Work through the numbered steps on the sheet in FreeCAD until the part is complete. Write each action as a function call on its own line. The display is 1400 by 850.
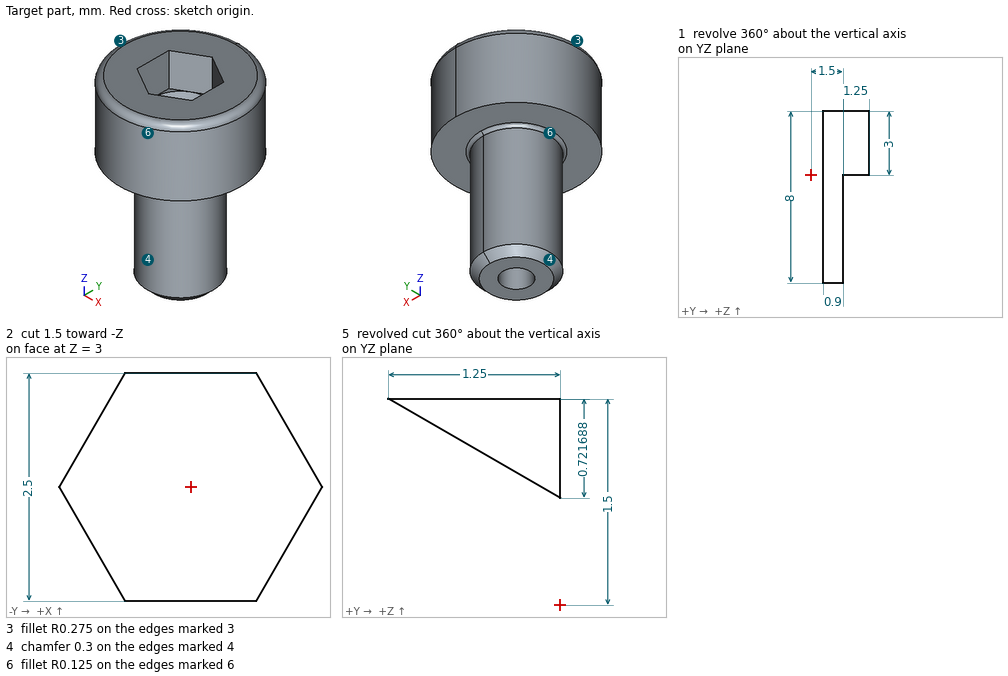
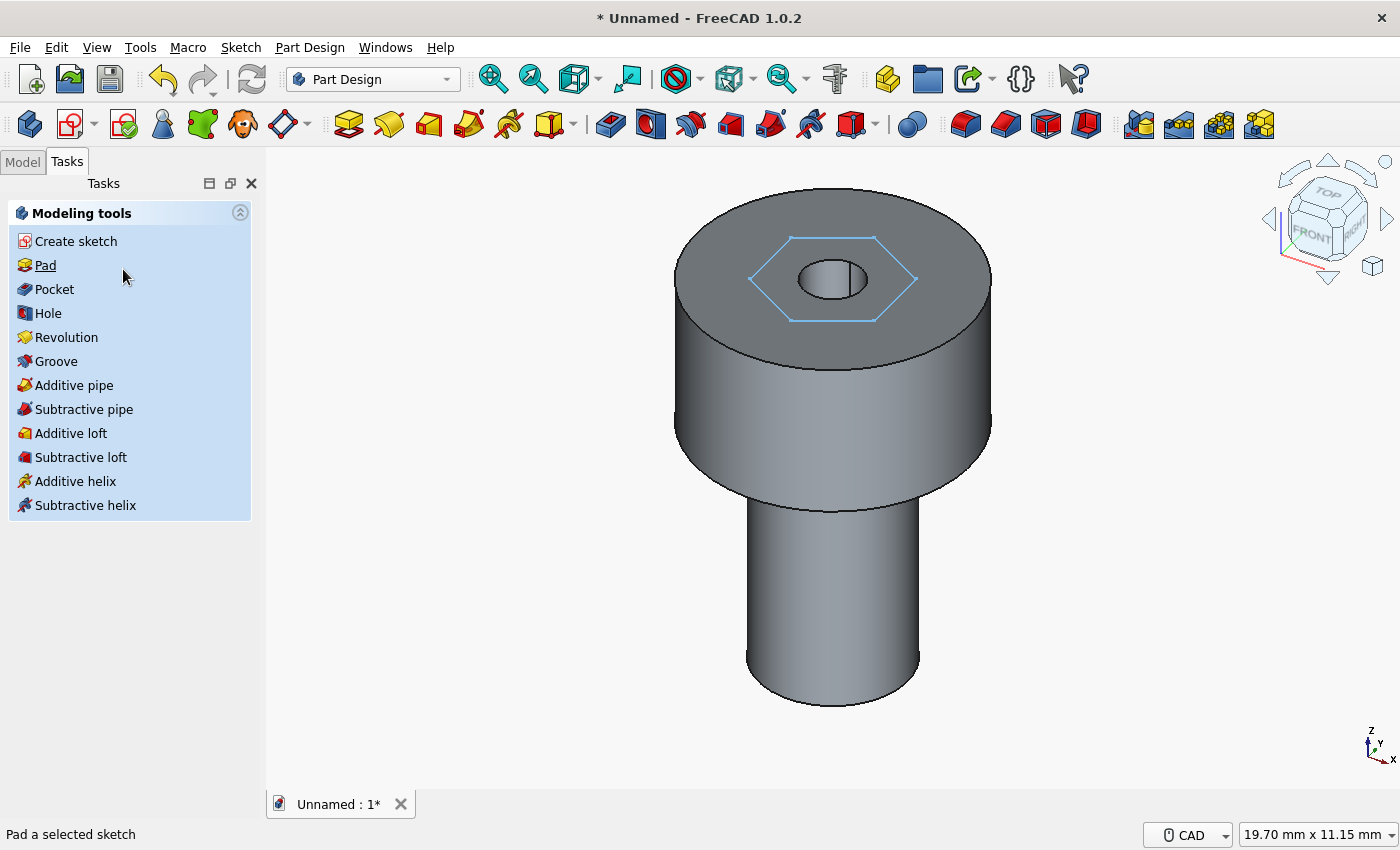
click(612, 124)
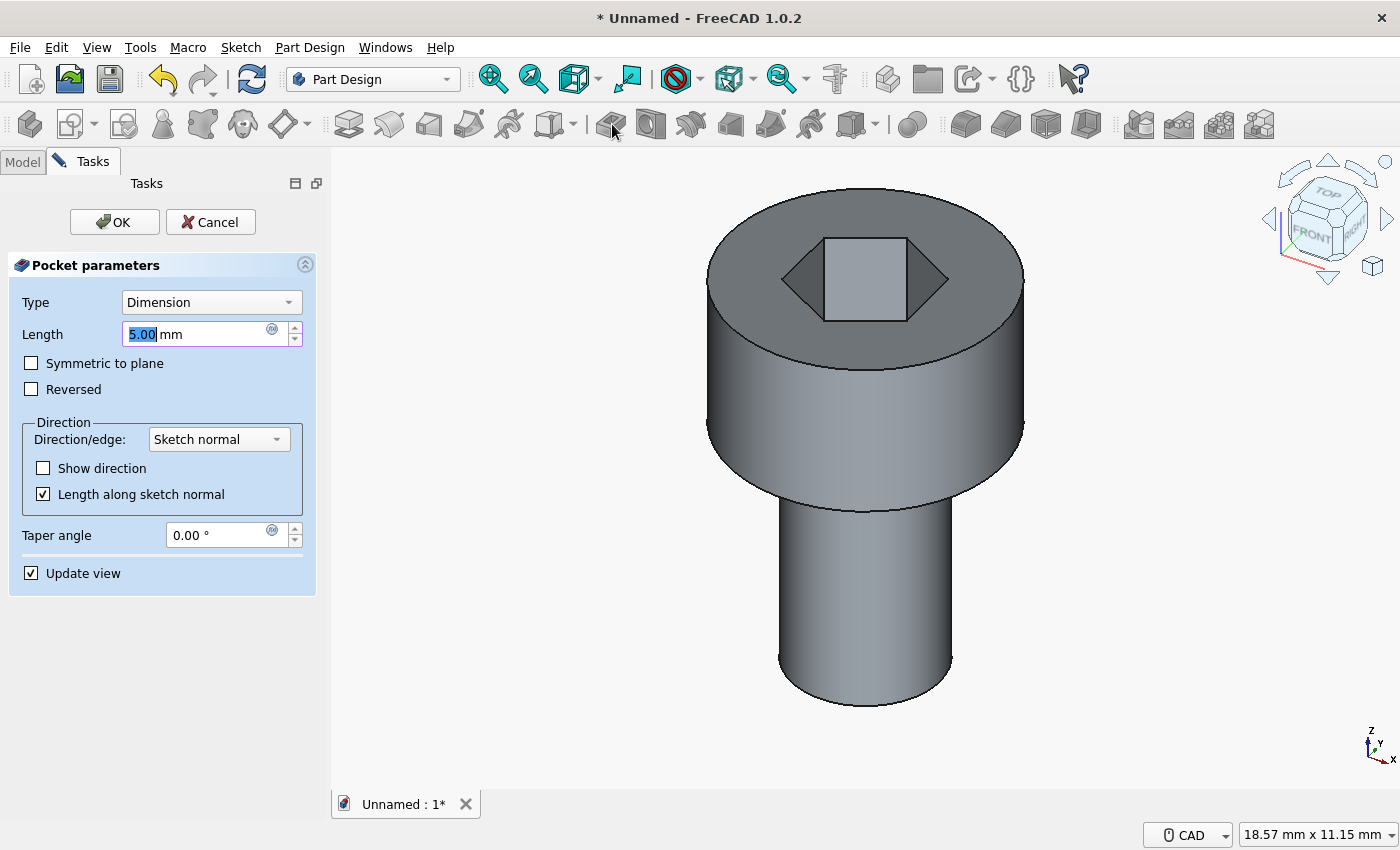
text(1.5)
key(Tab)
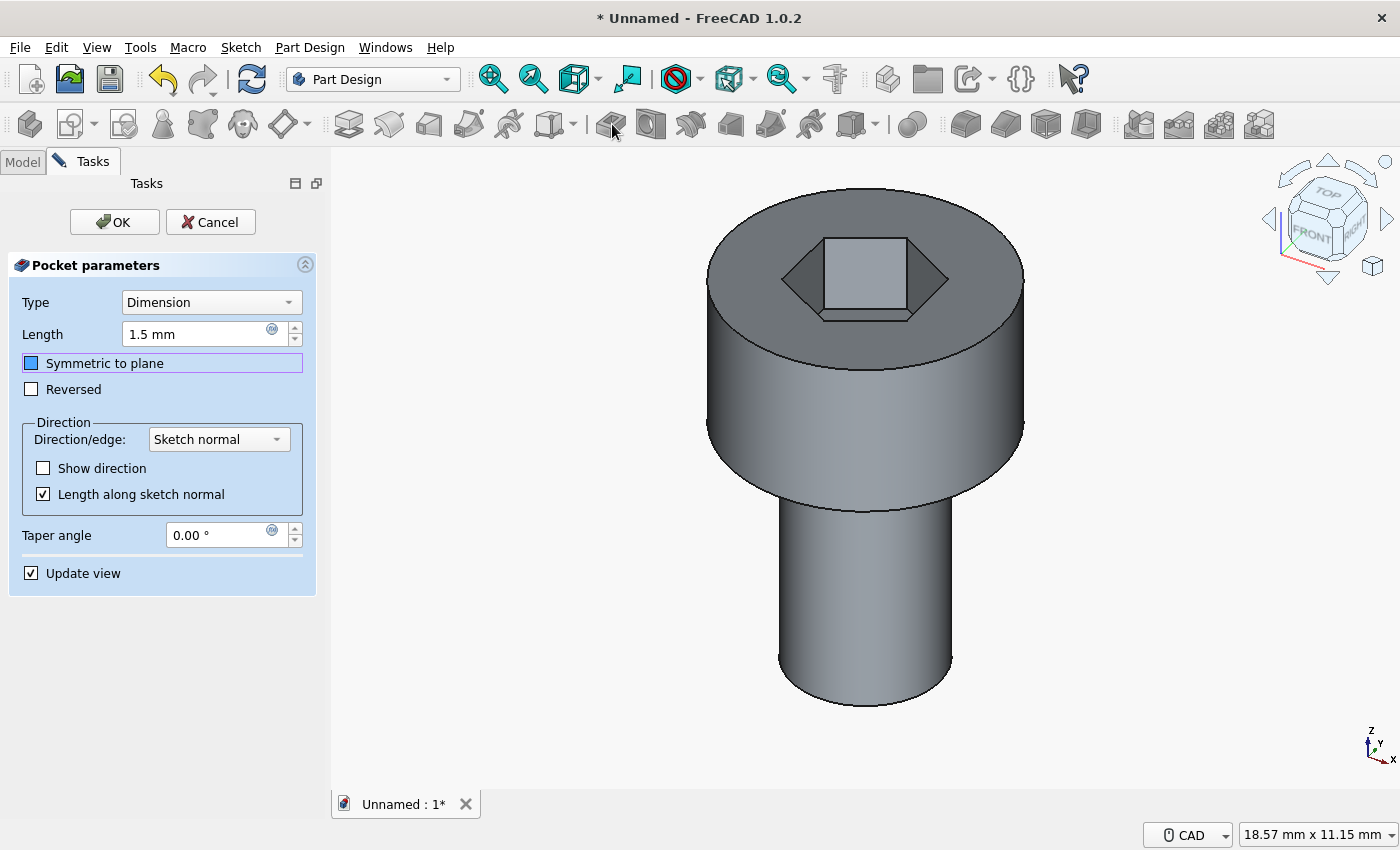
click(115, 222)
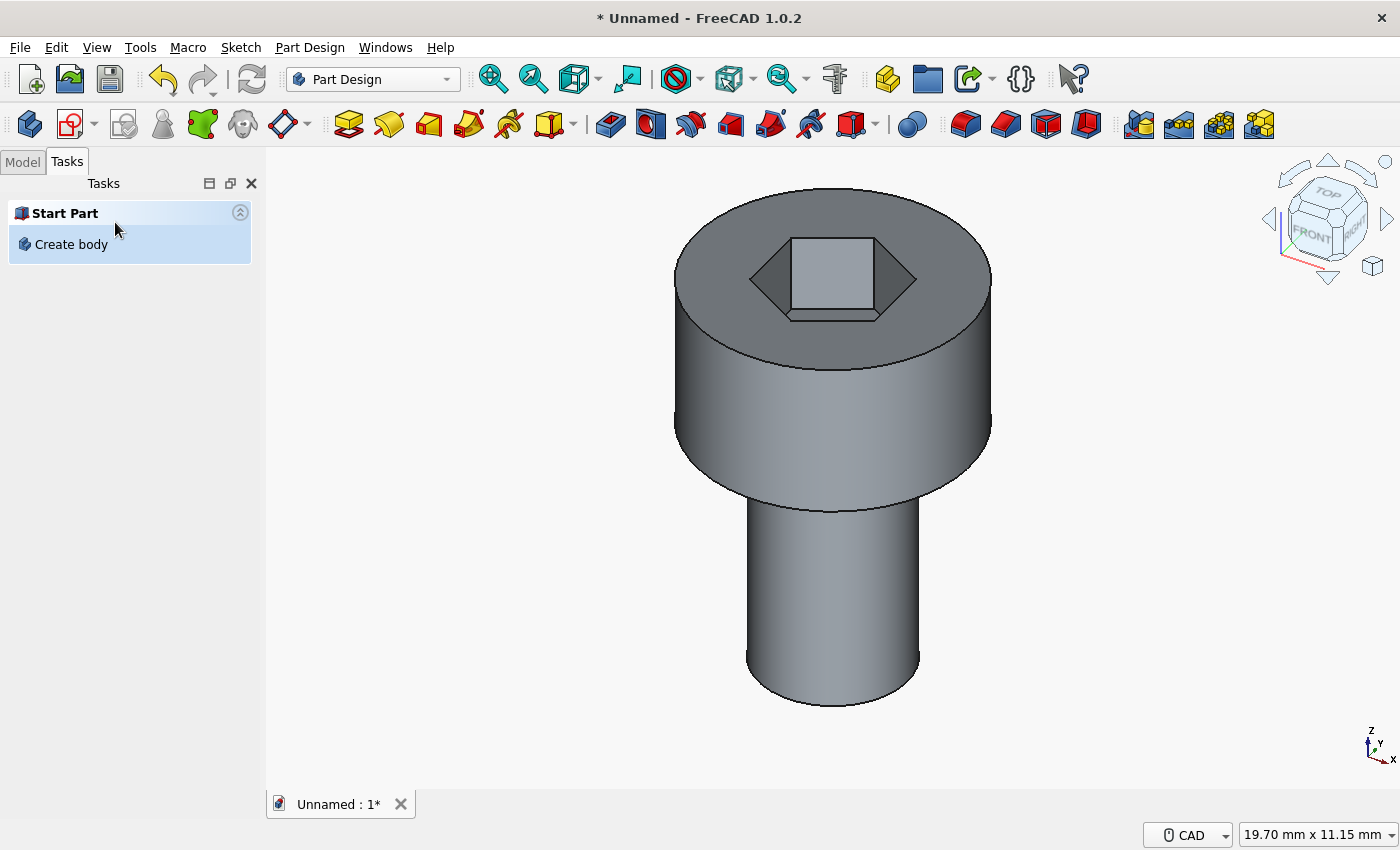
click(754, 357)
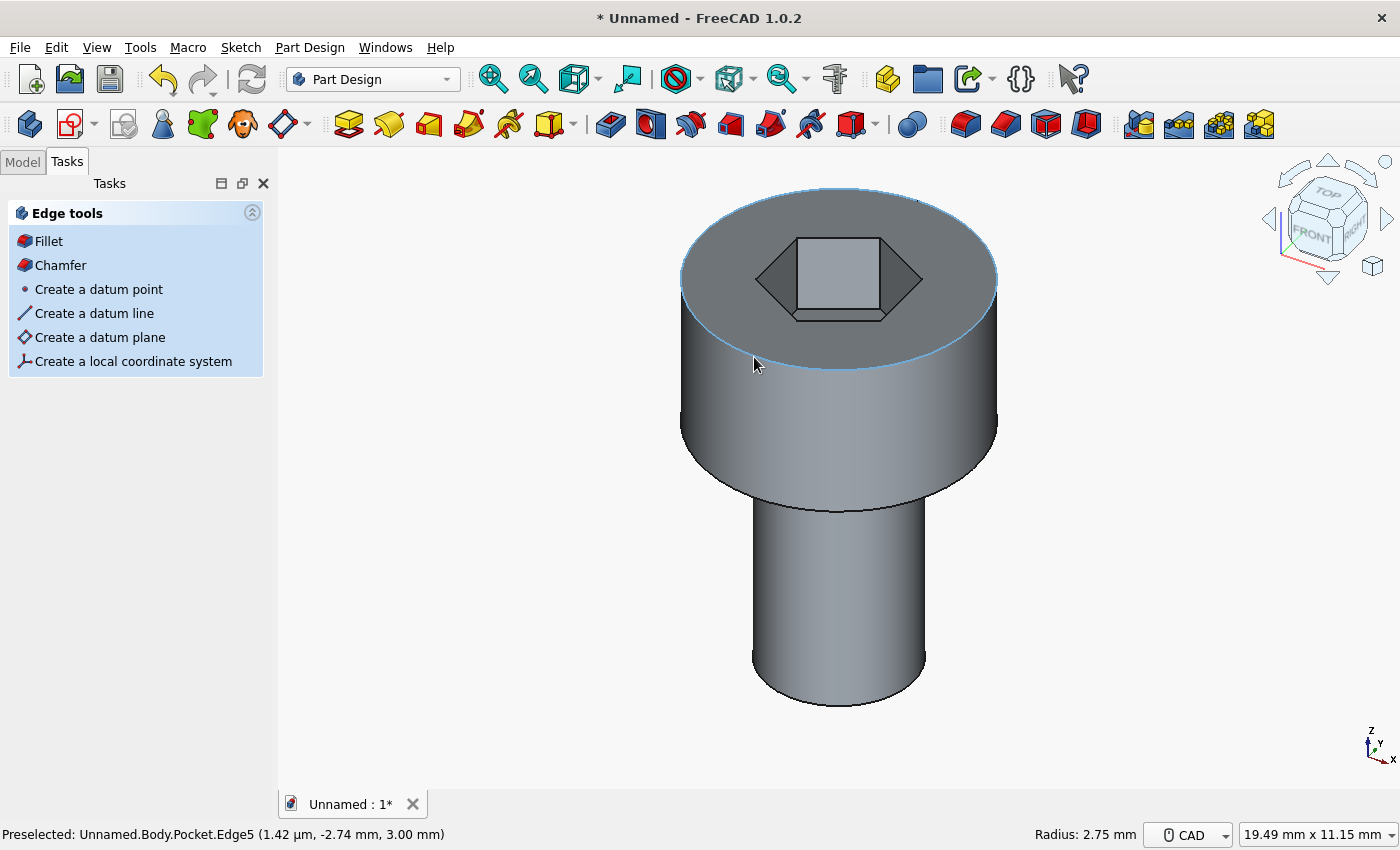
click(966, 124)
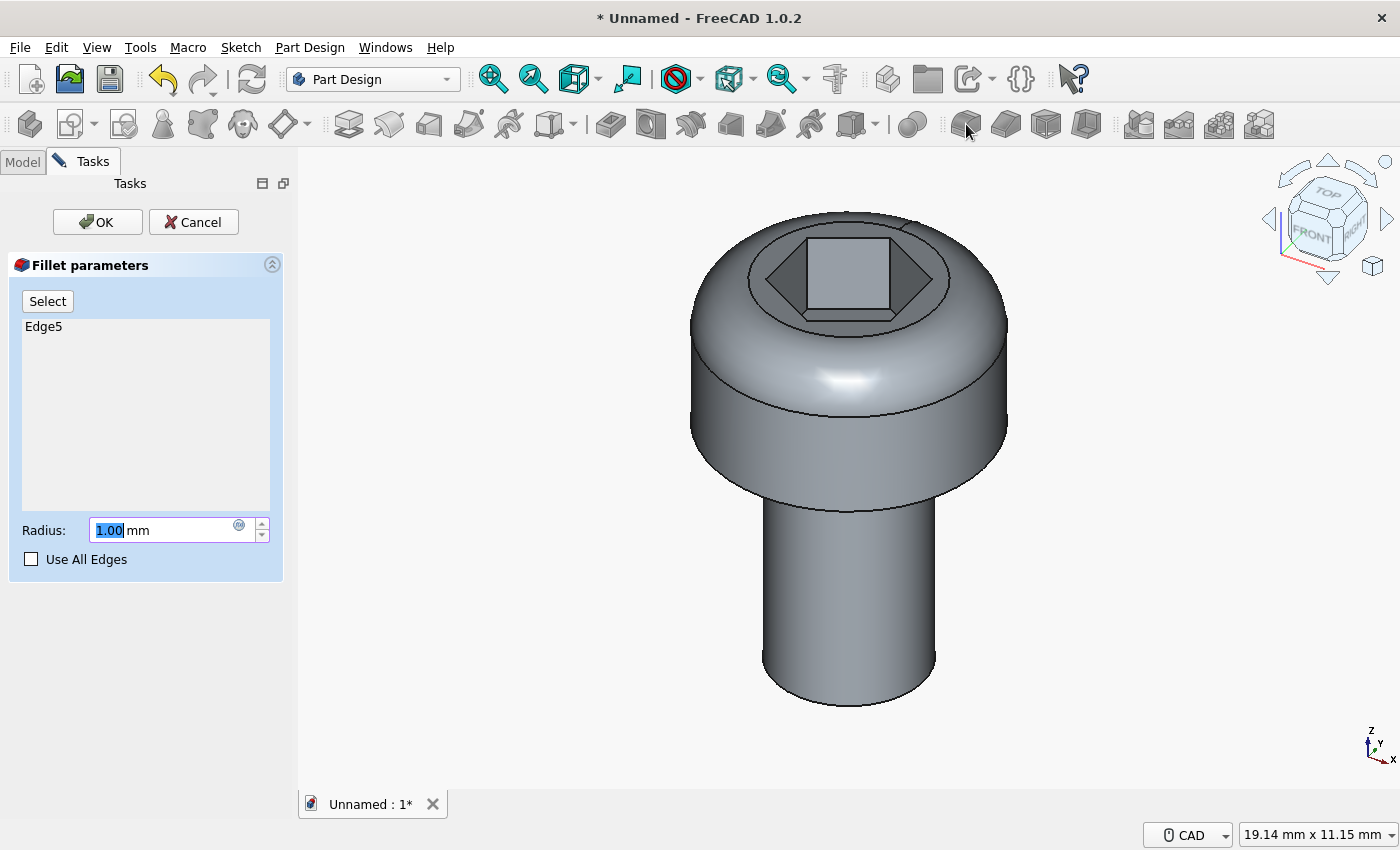
text(0.275)
key(Tab)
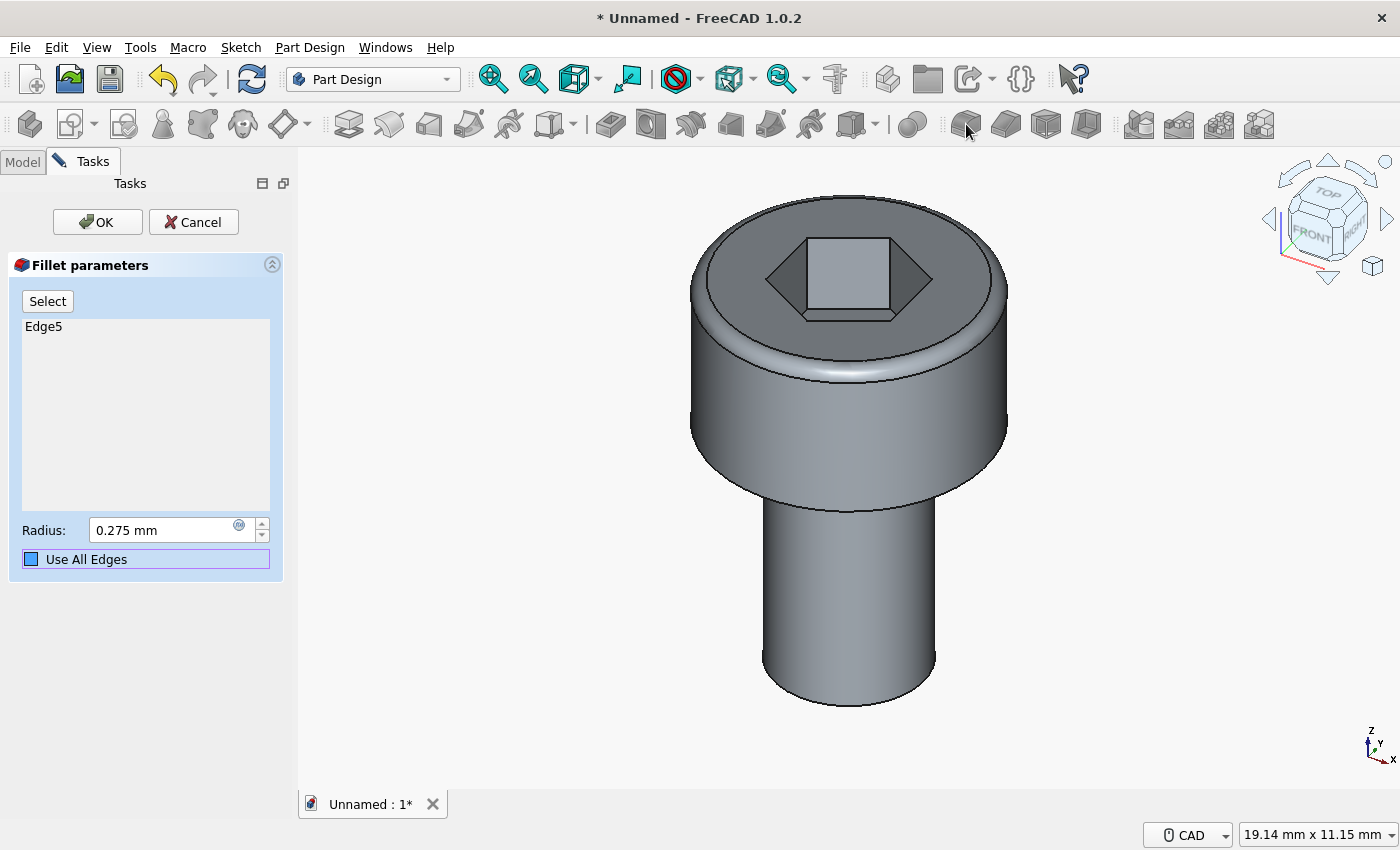
click(98, 222)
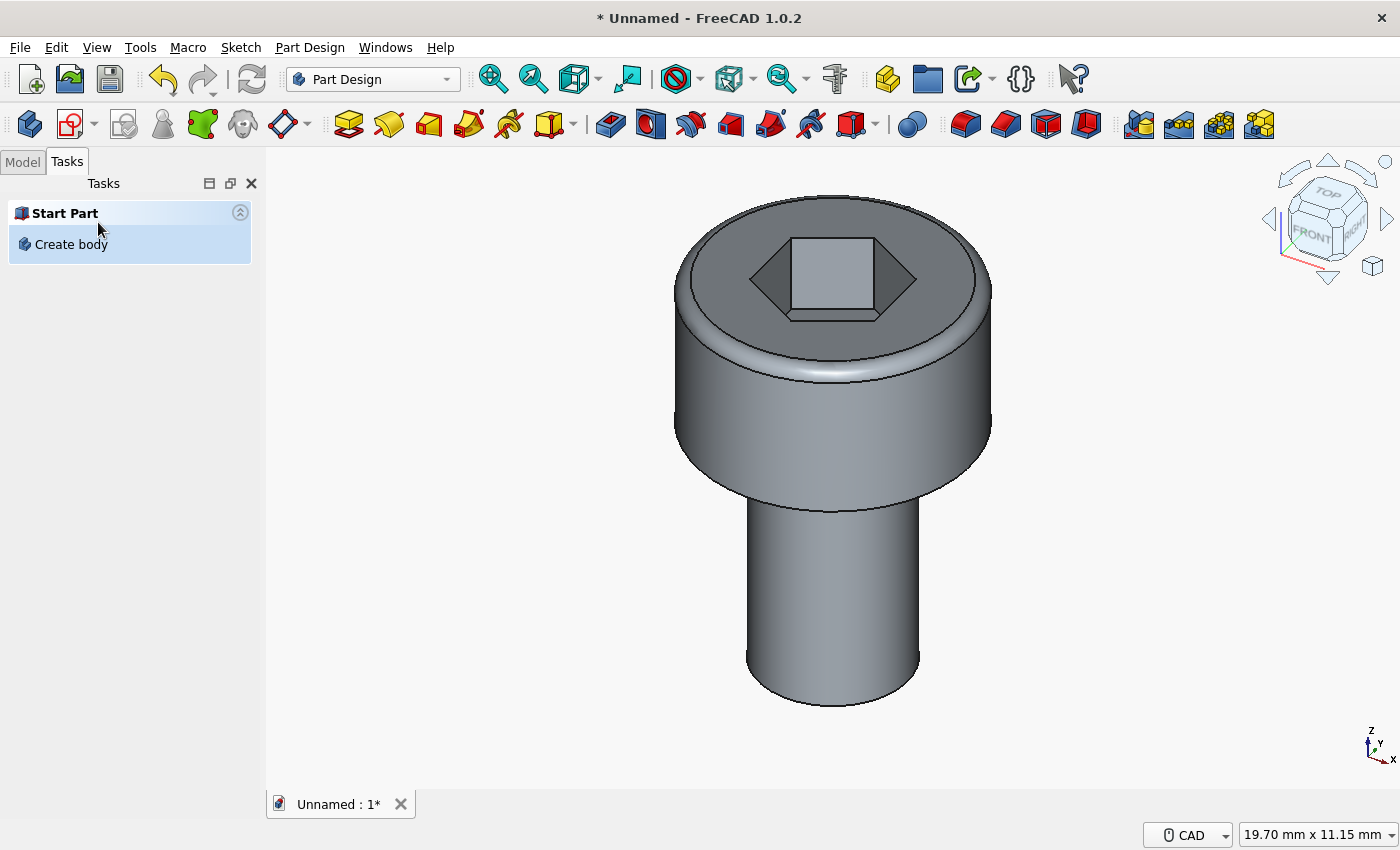
key(0)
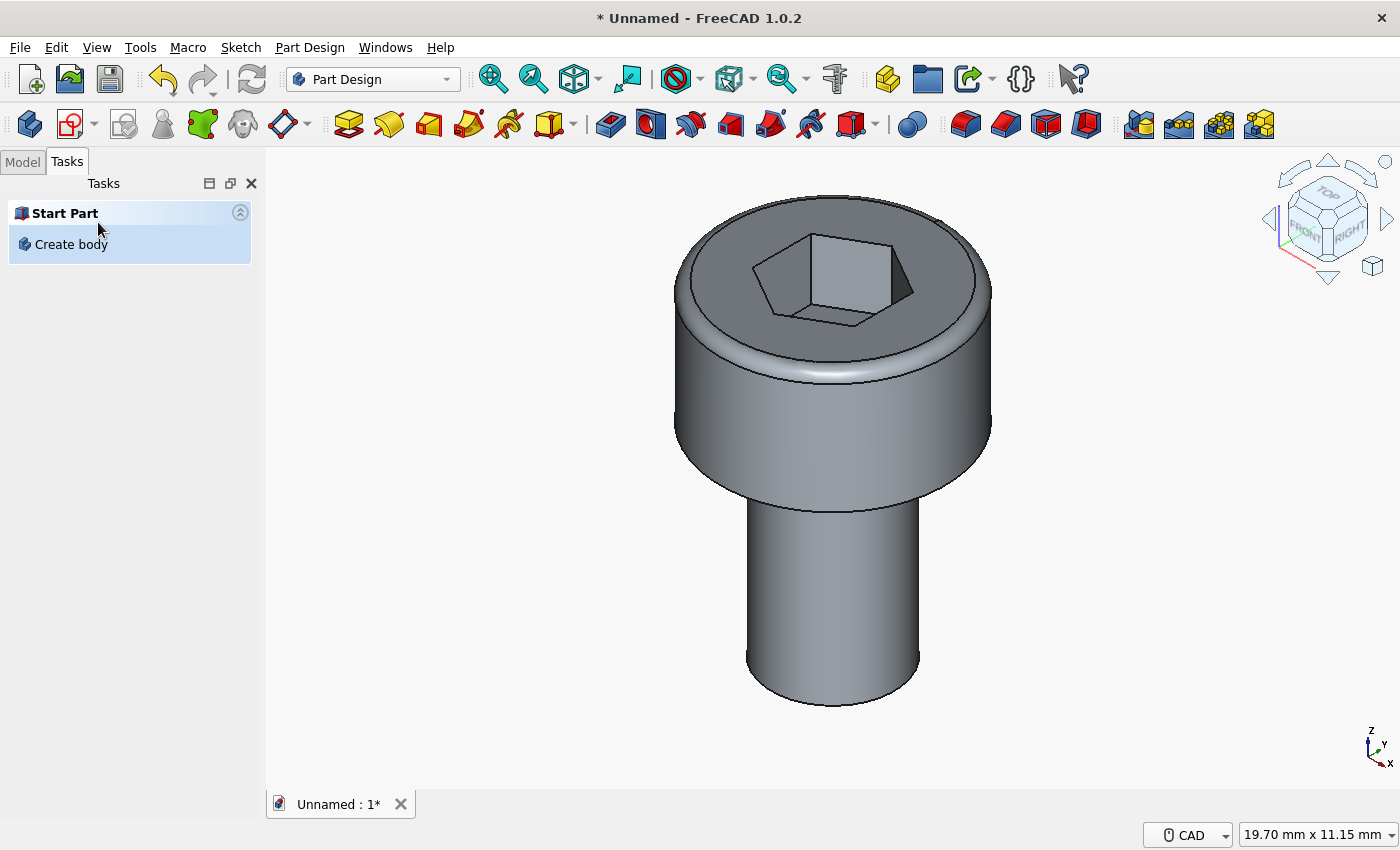
key(2)